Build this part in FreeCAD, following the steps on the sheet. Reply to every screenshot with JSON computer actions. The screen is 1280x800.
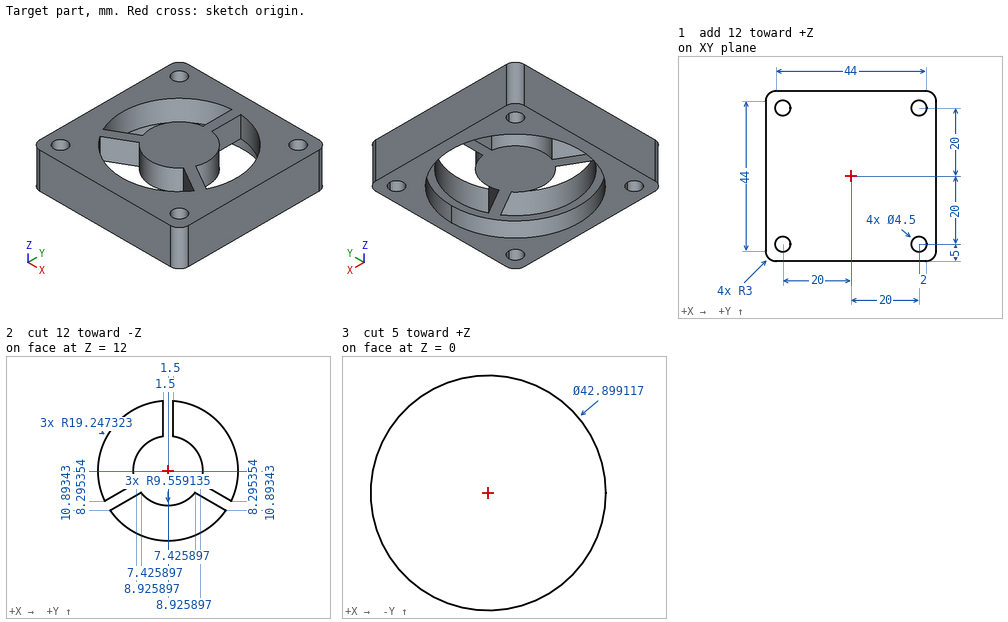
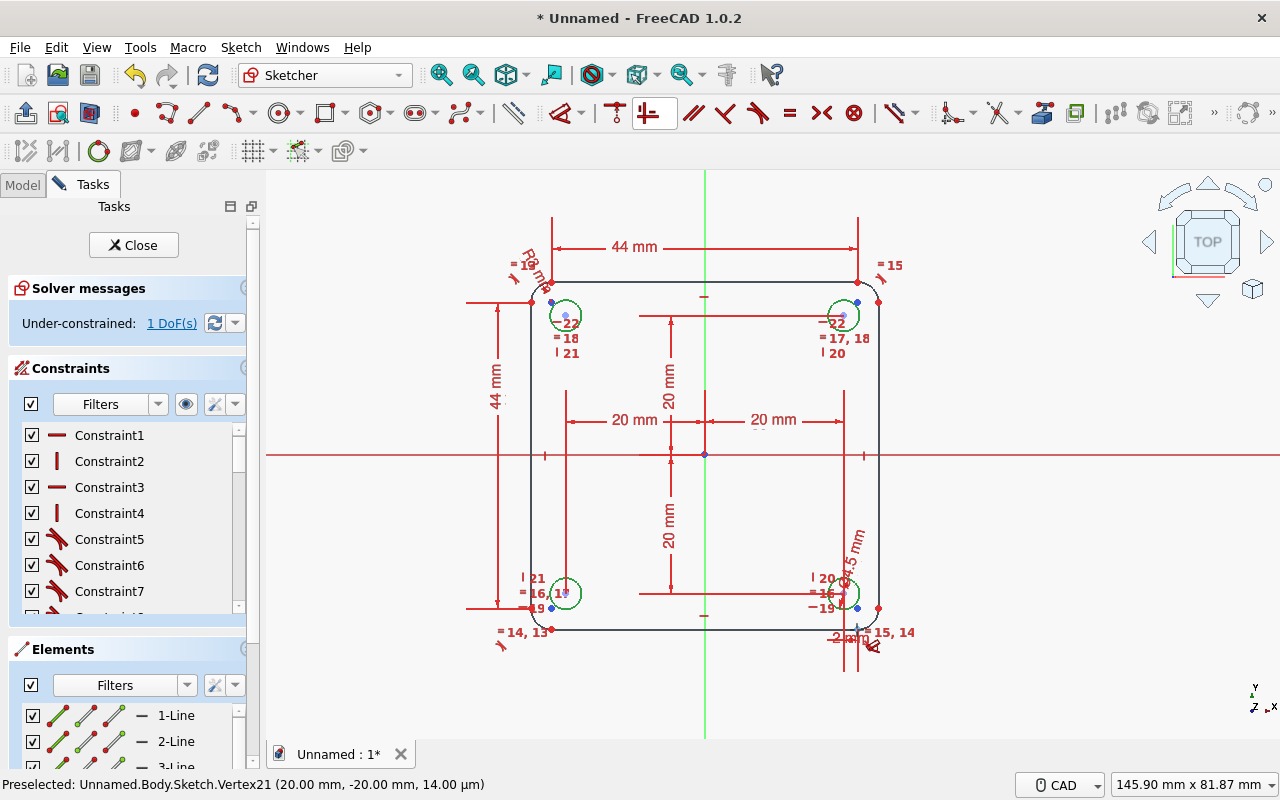
{"action": "left_click", "coordinate": [858, 630]}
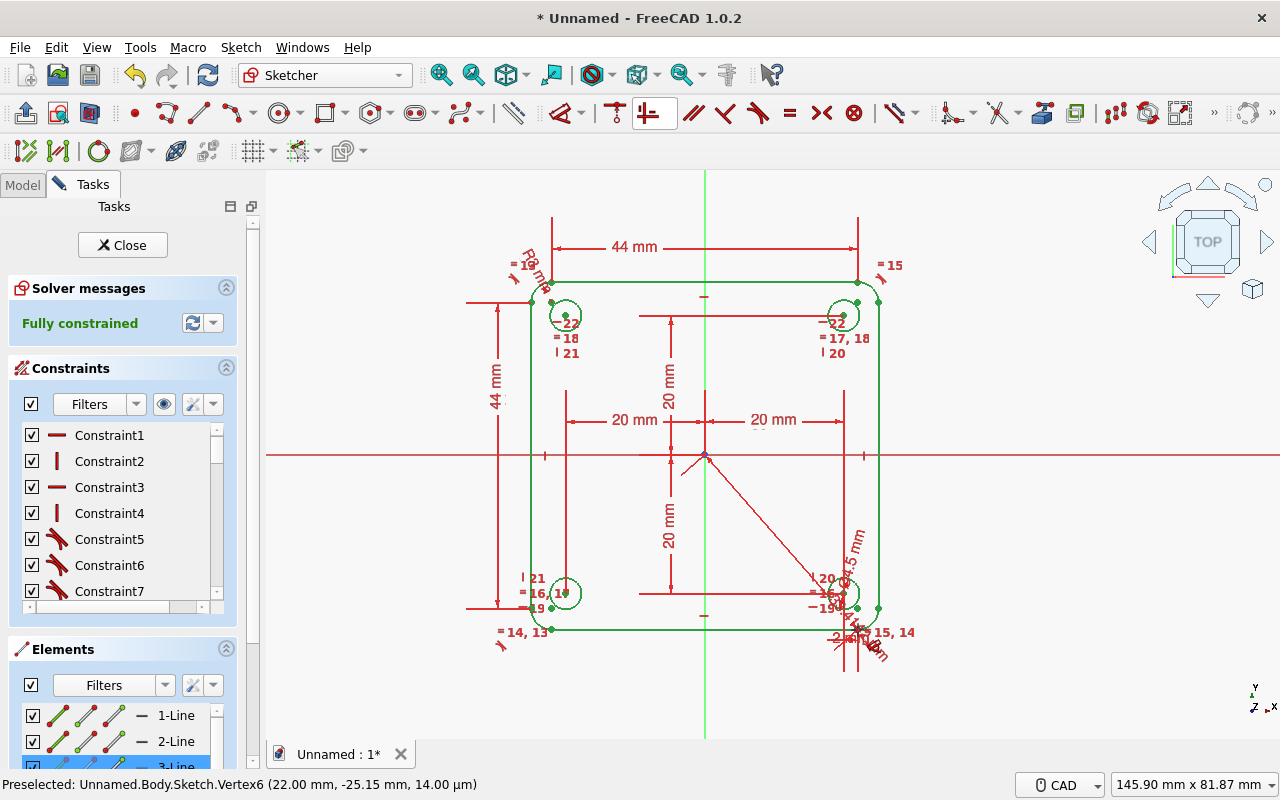
{"action": "left_click", "coordinate": [844, 594]}
{"action": "left_click", "coordinate": [892, 612]}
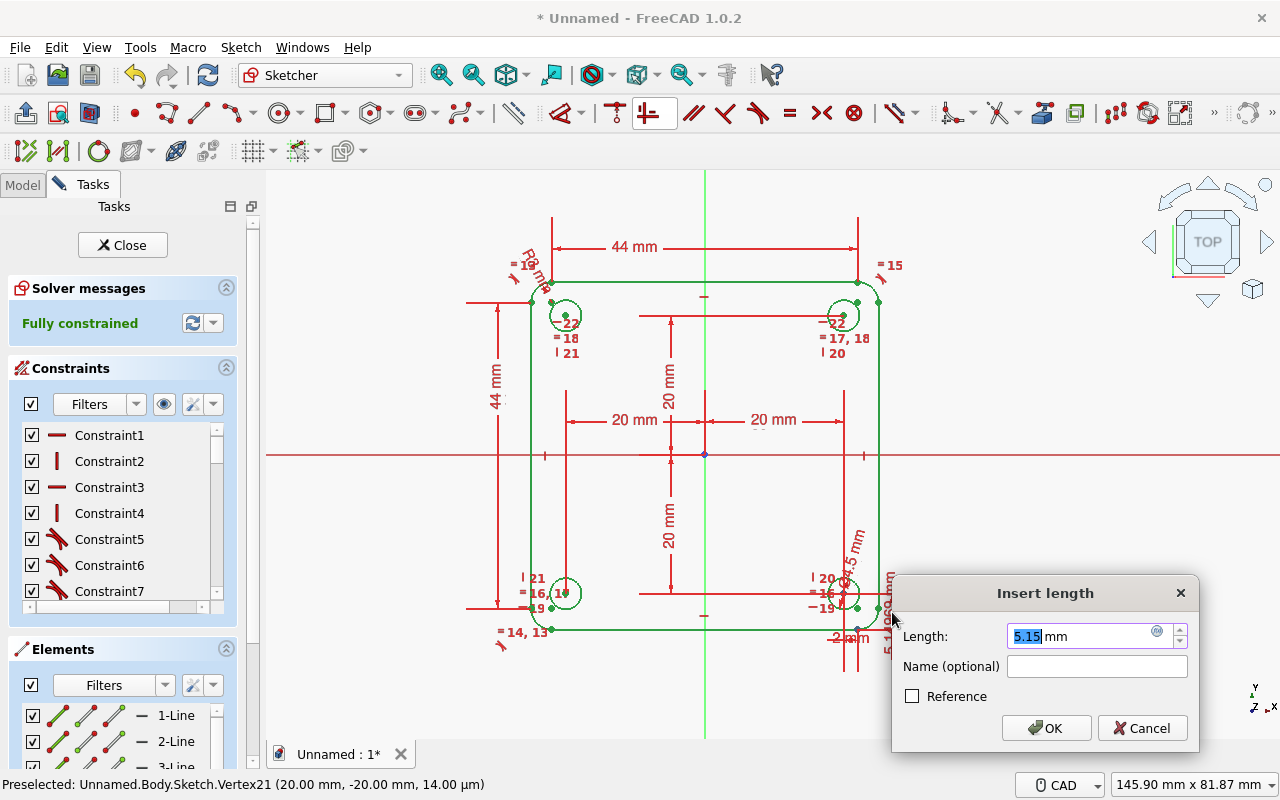
{"action": "type", "text": "5"}
{"action": "key", "text": "Return"}
{"action": "key", "text": "Escape"}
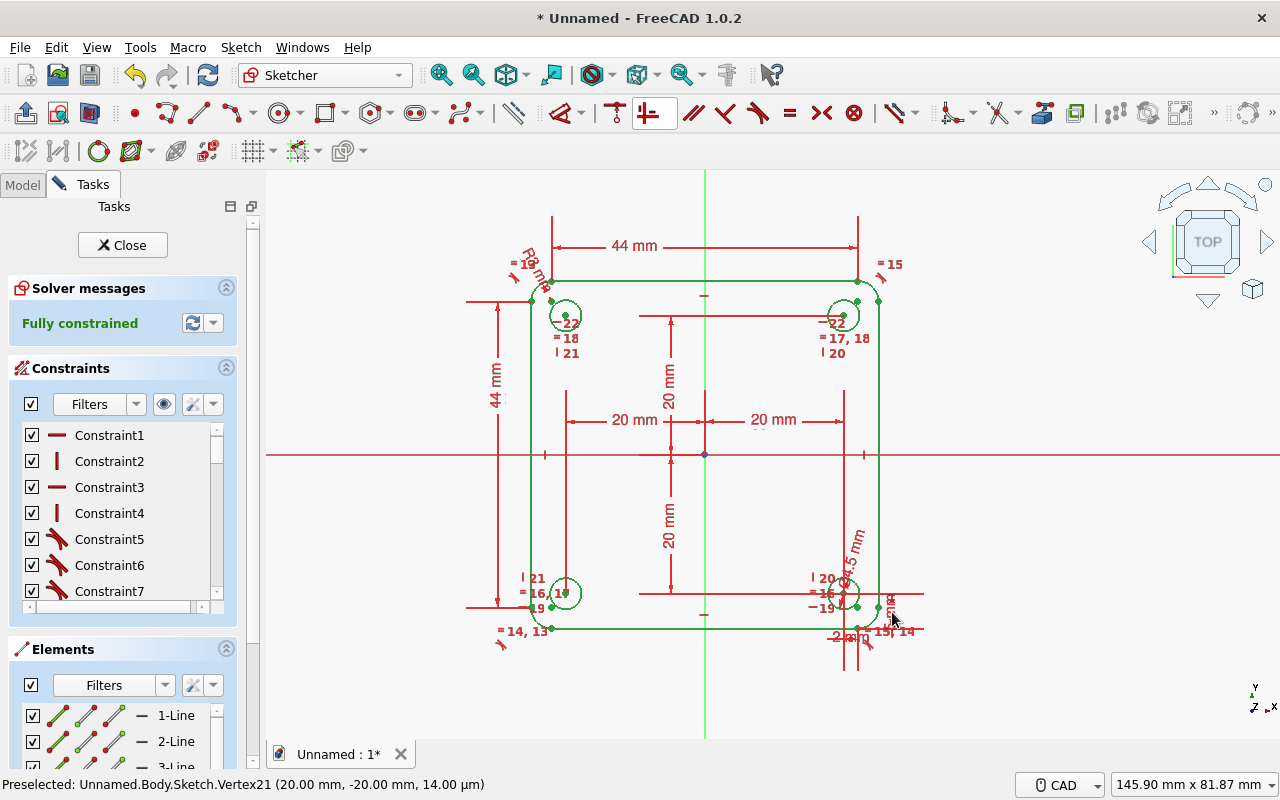
{"action": "left_click", "coordinate": [123, 245]}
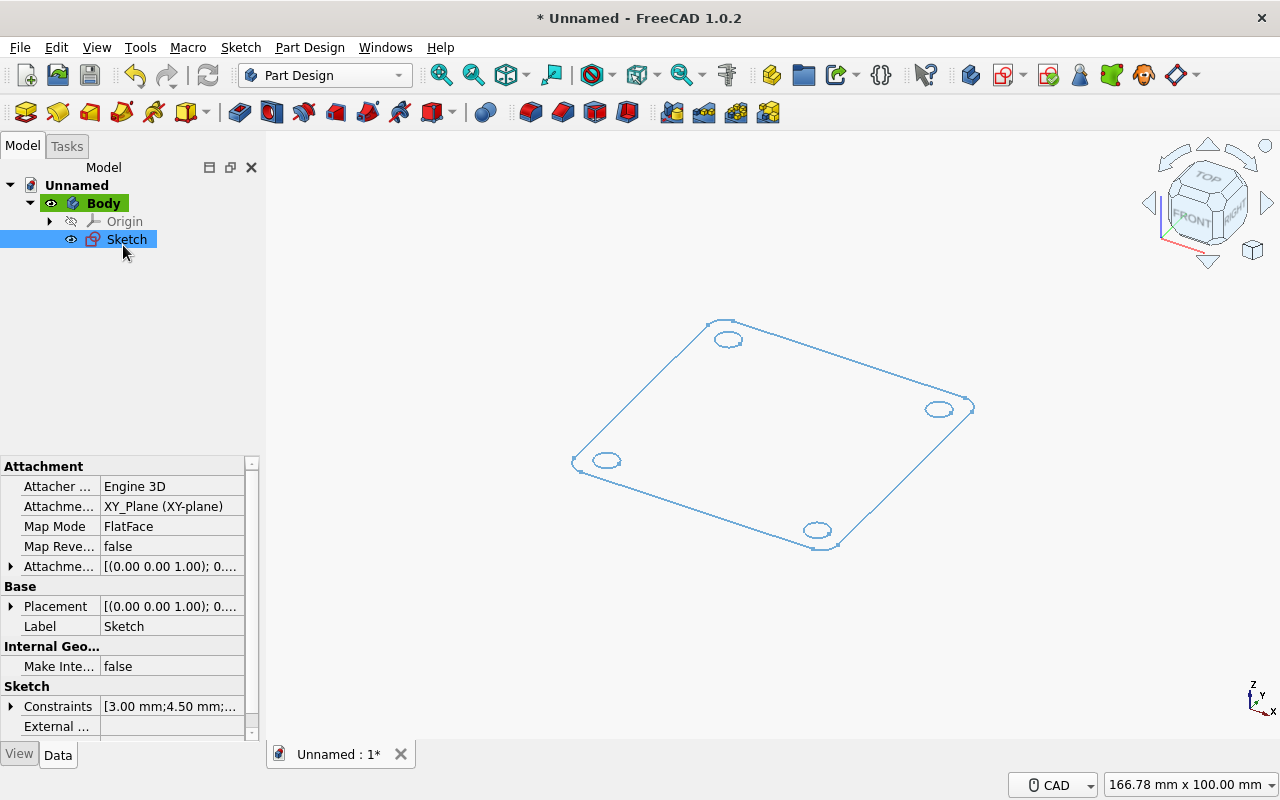
{"action": "left_click", "coordinate": [26, 112]}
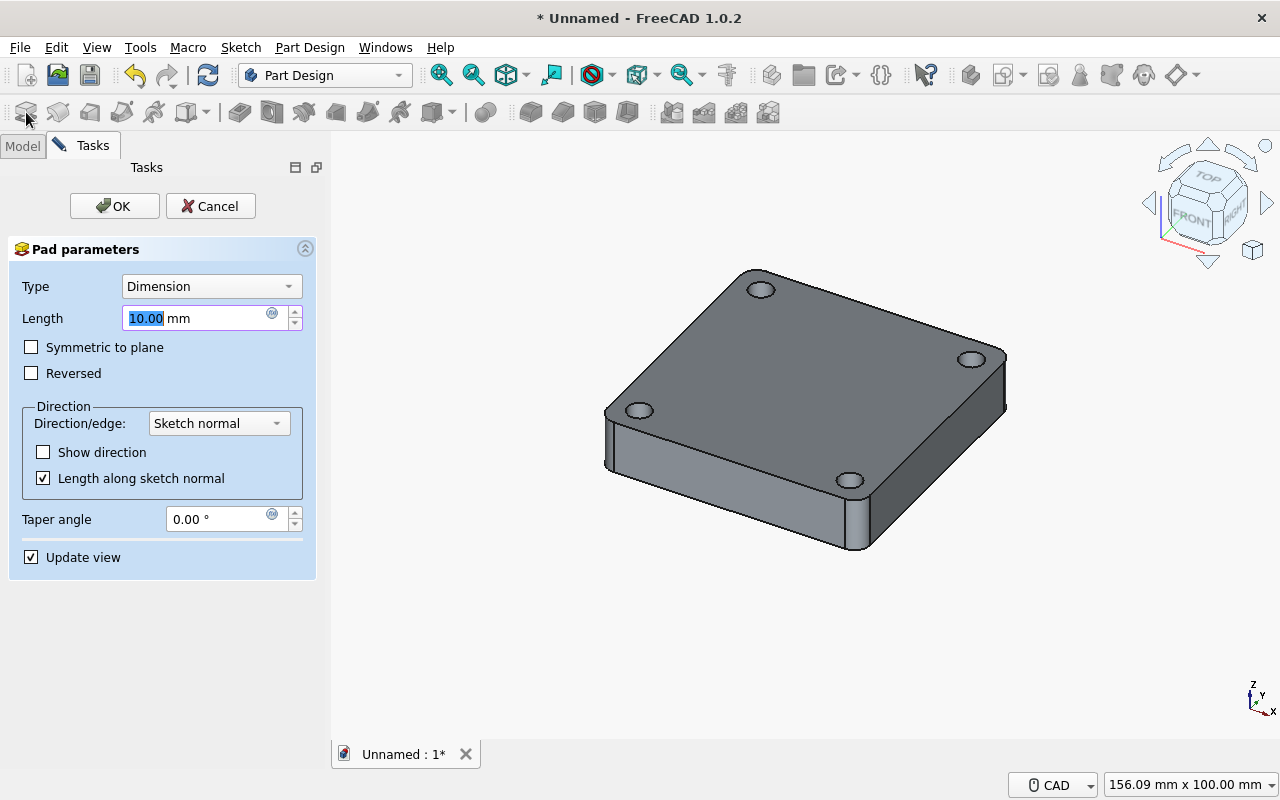
{"action": "type", "text": "12"}
{"action": "key", "text": "Tab"}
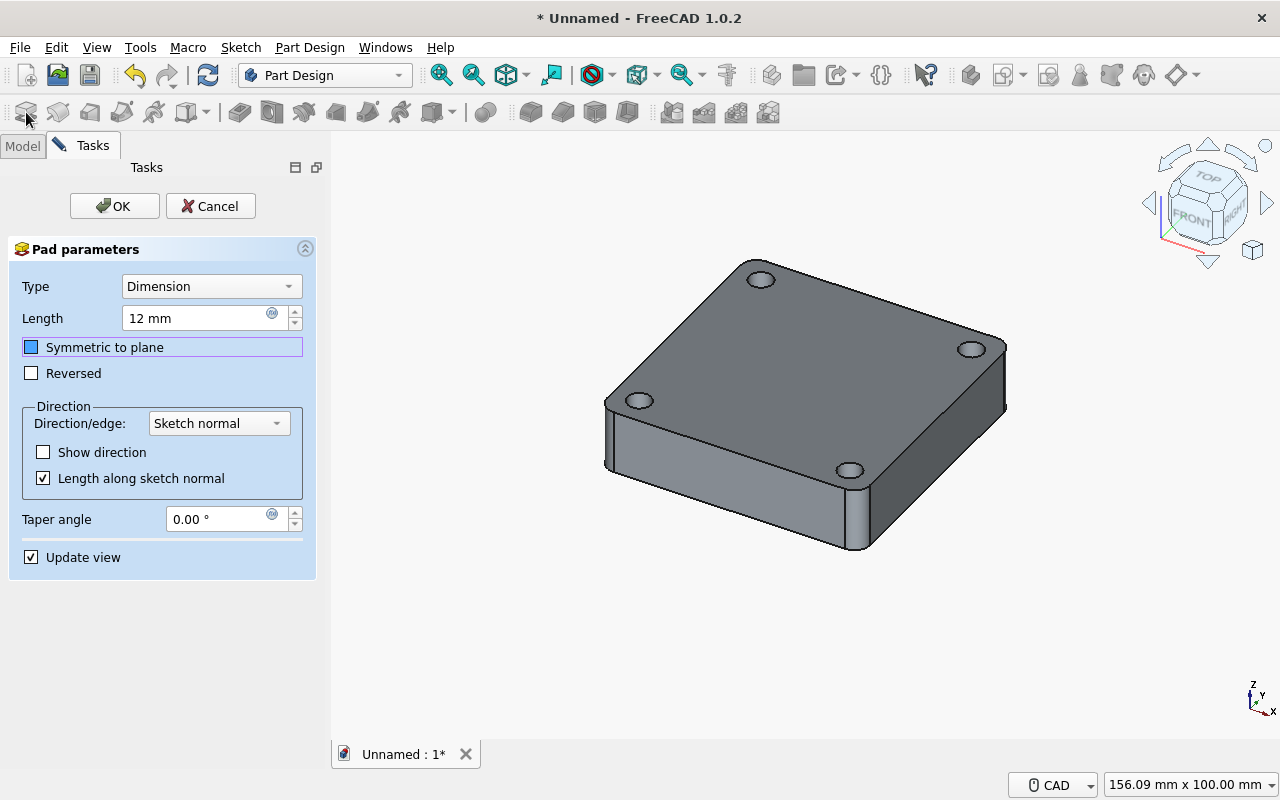
{"action": "left_click", "coordinate": [115, 206]}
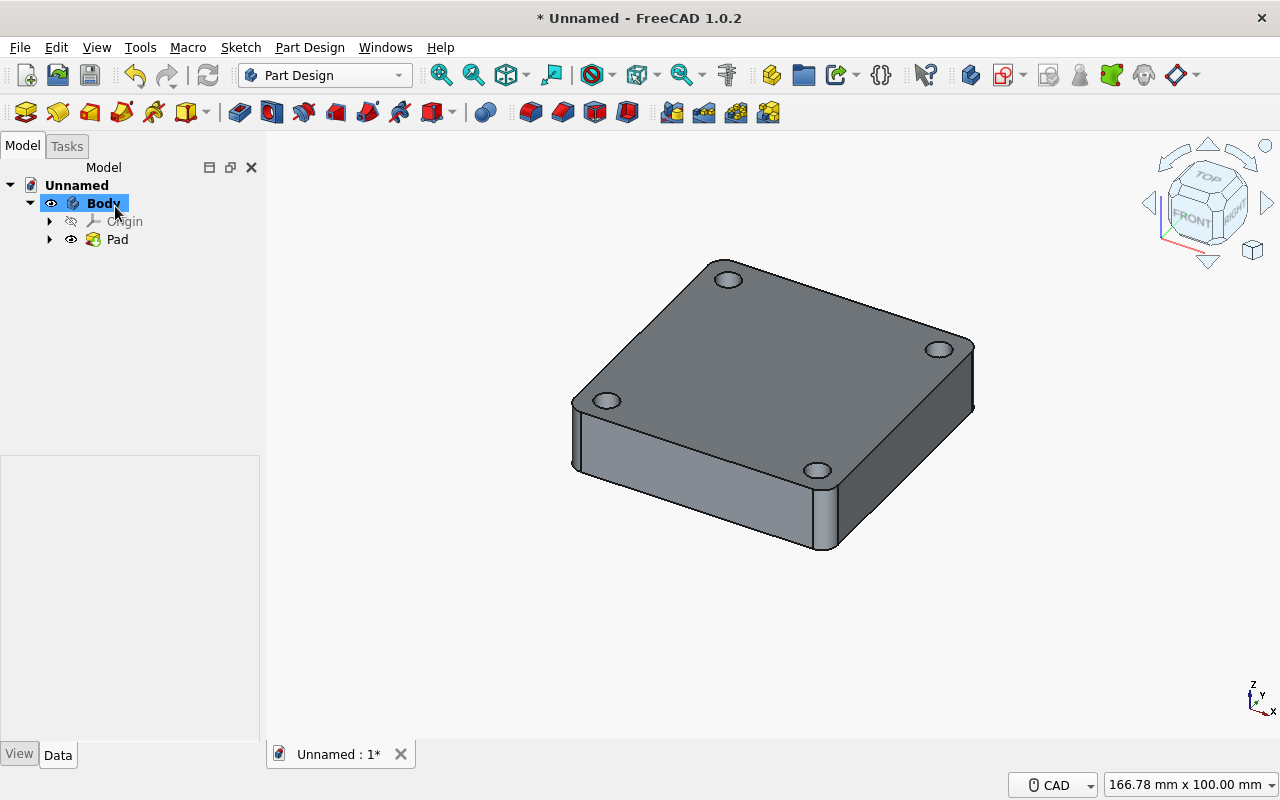
{"action": "left_click", "coordinate": [773, 374]}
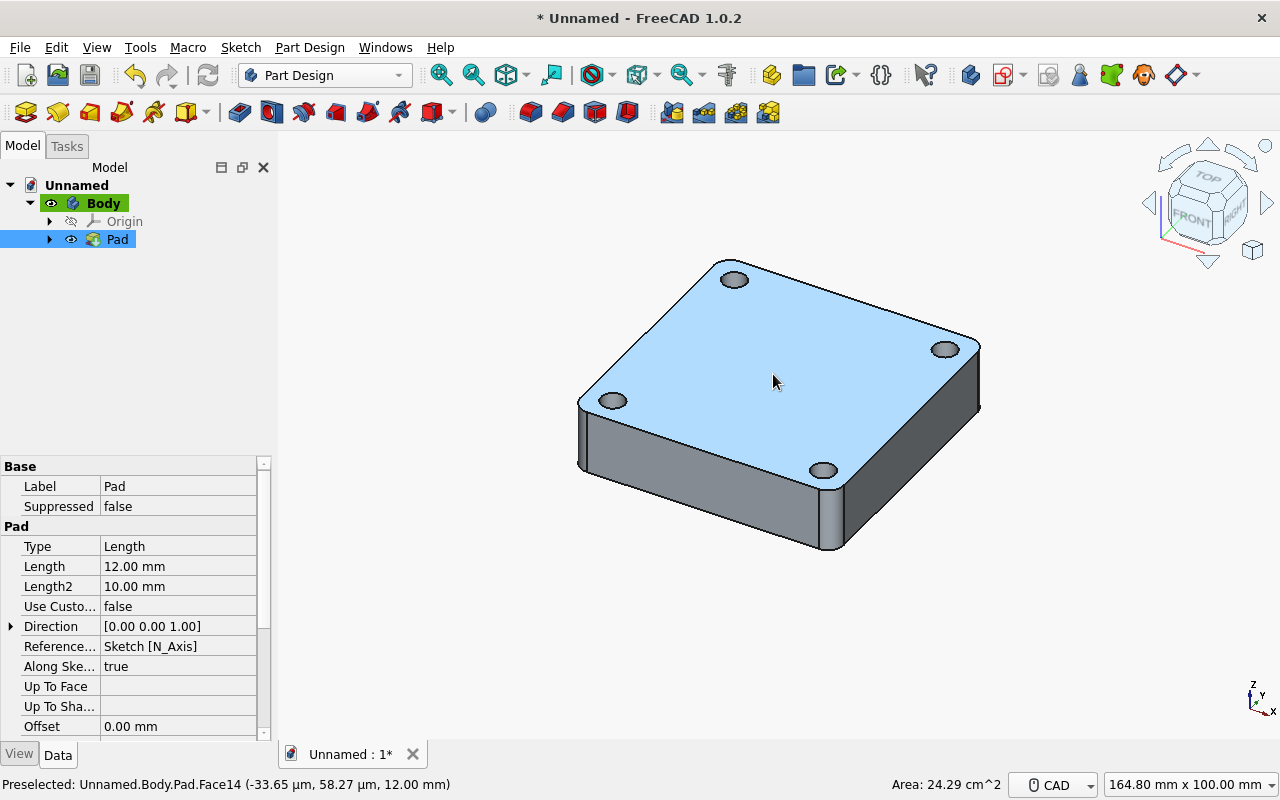
{"action": "left_click", "coordinate": [1004, 76]}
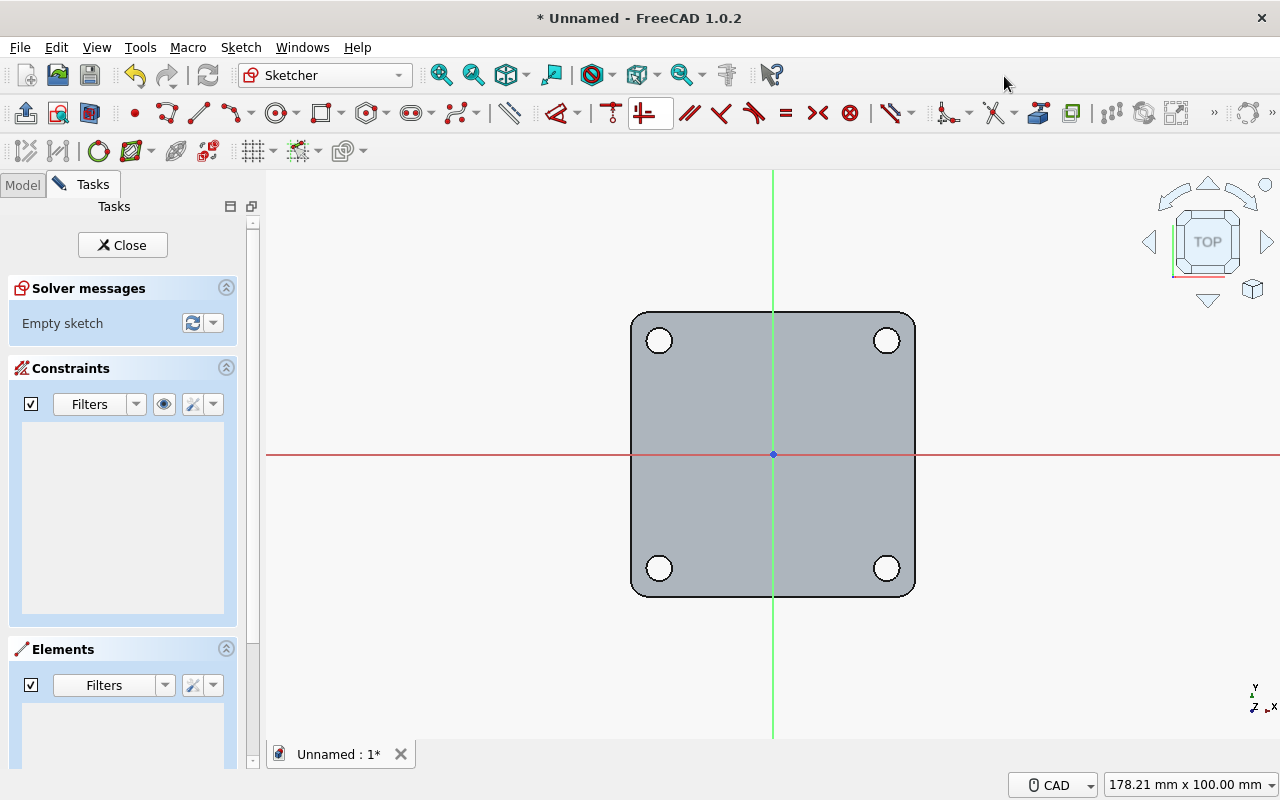
{"action": "scroll", "coordinate": [856, 455], "scroll_direction": "up", "scroll_amount": 3}